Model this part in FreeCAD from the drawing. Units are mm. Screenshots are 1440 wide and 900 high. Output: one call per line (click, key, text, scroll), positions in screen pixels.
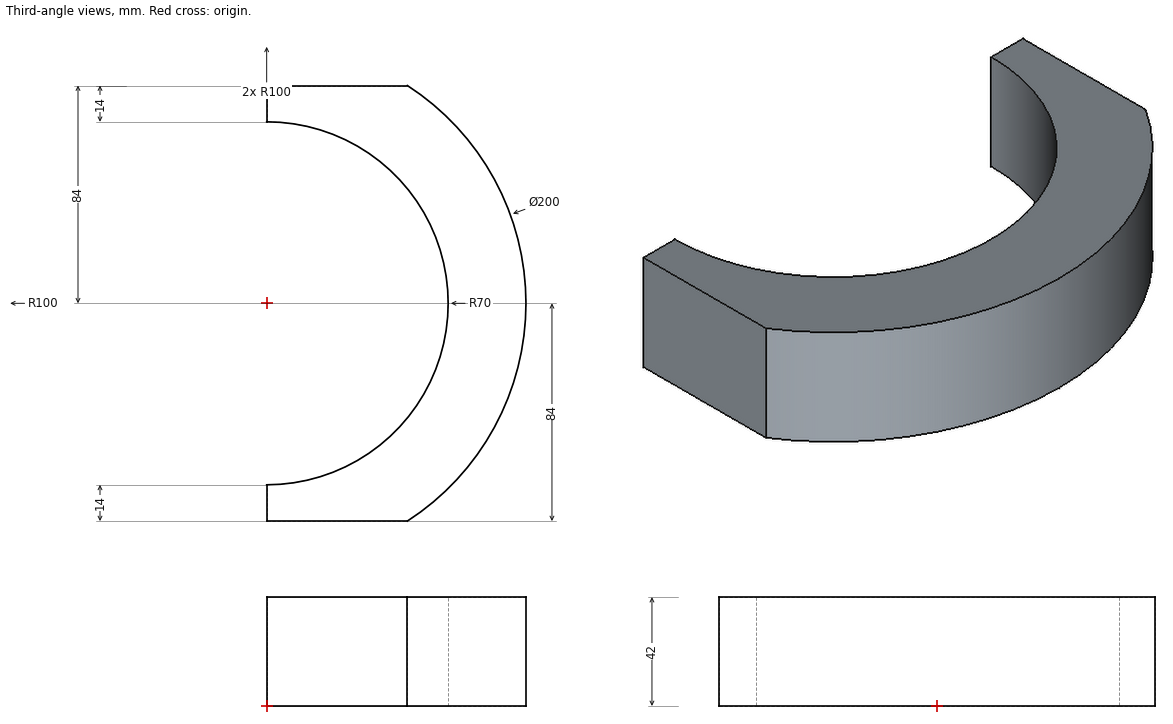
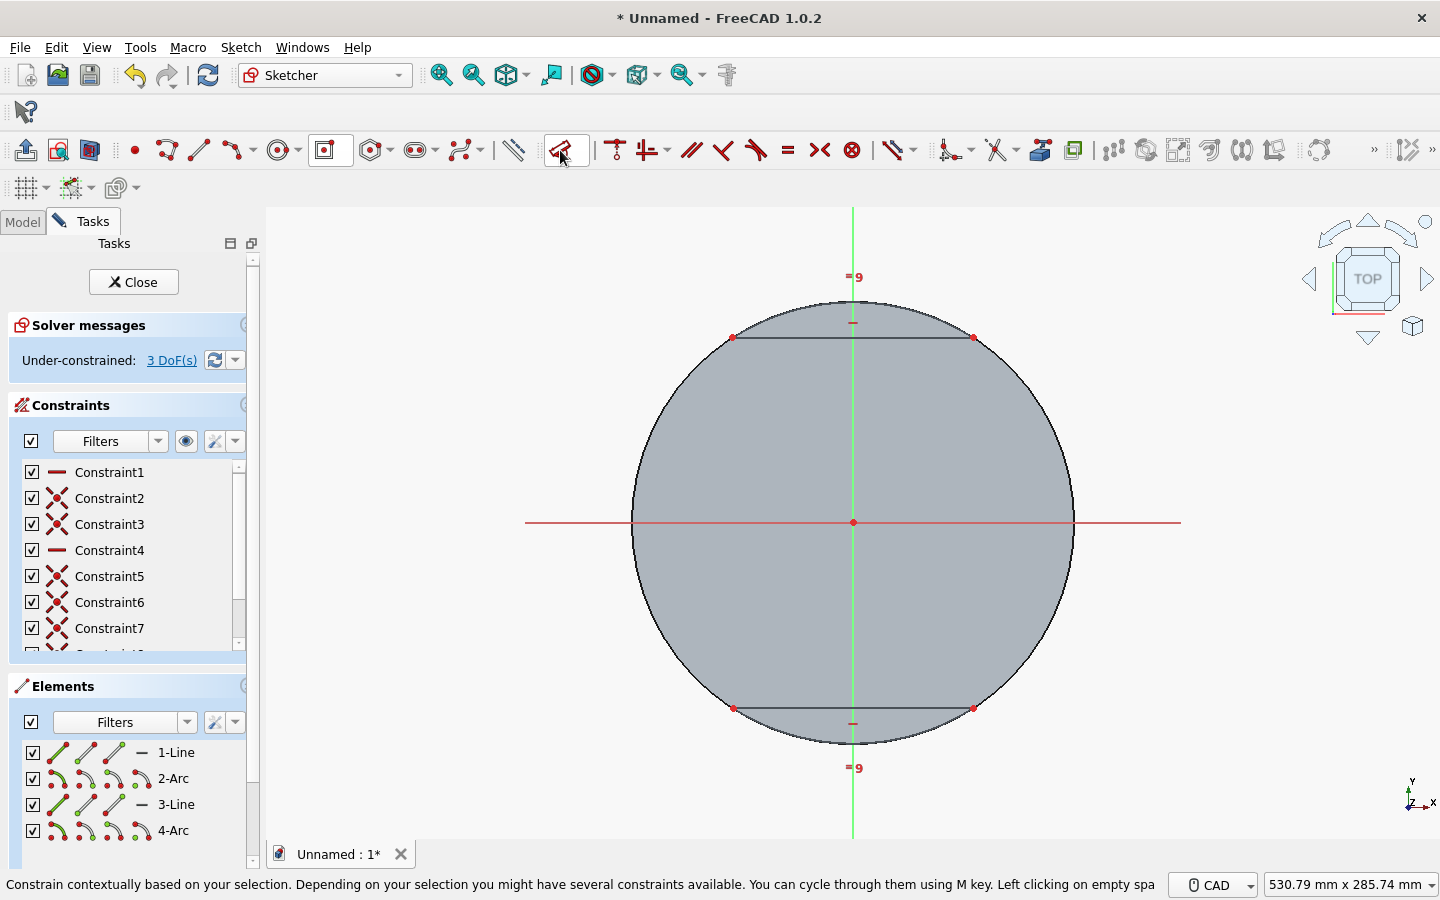
click(903, 308)
click(910, 277)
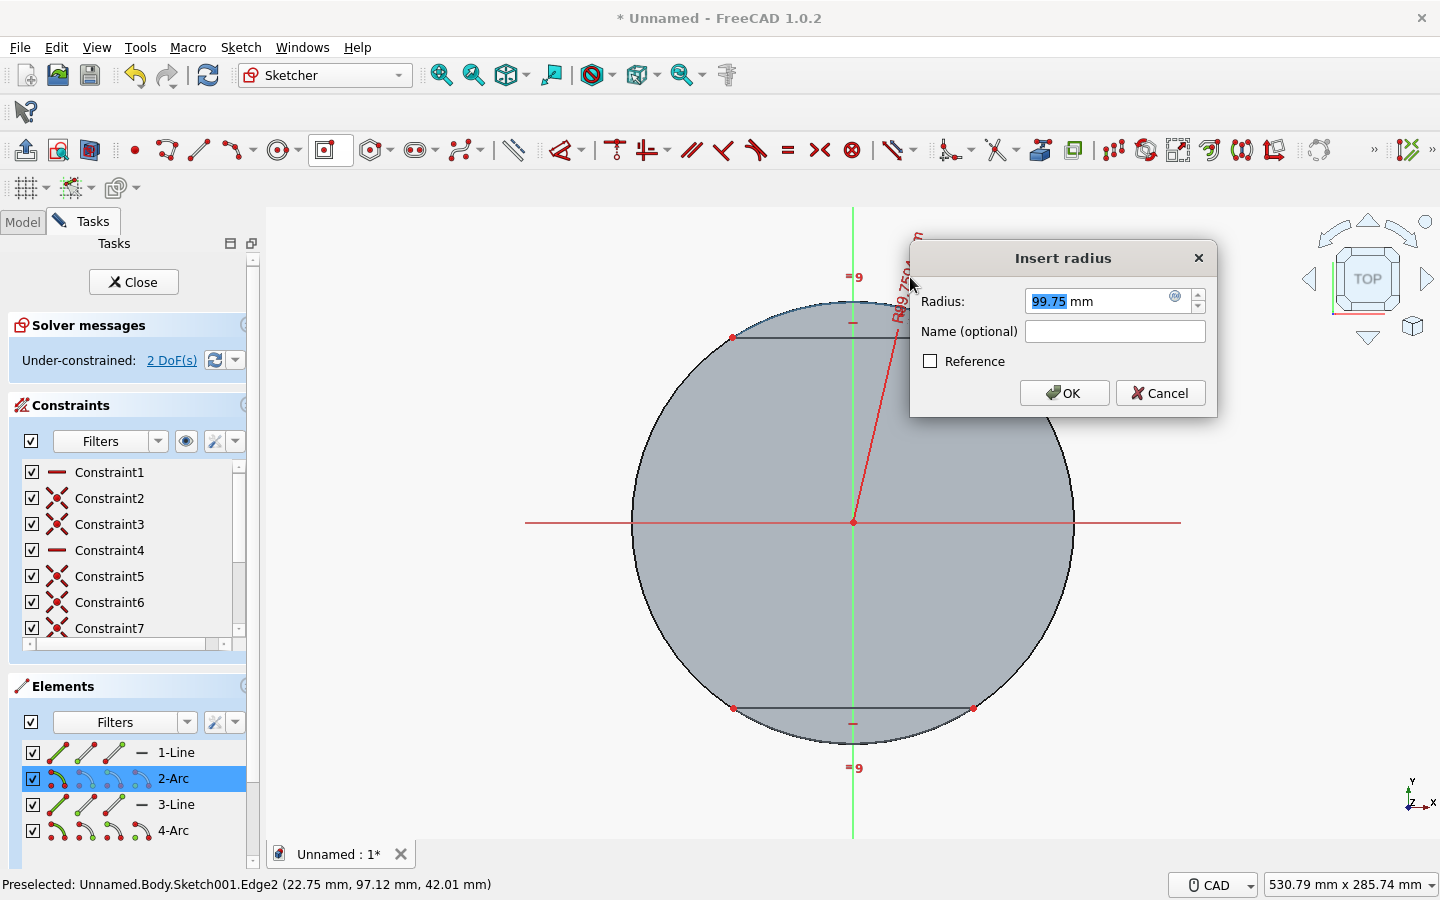
text(100)
key(Return)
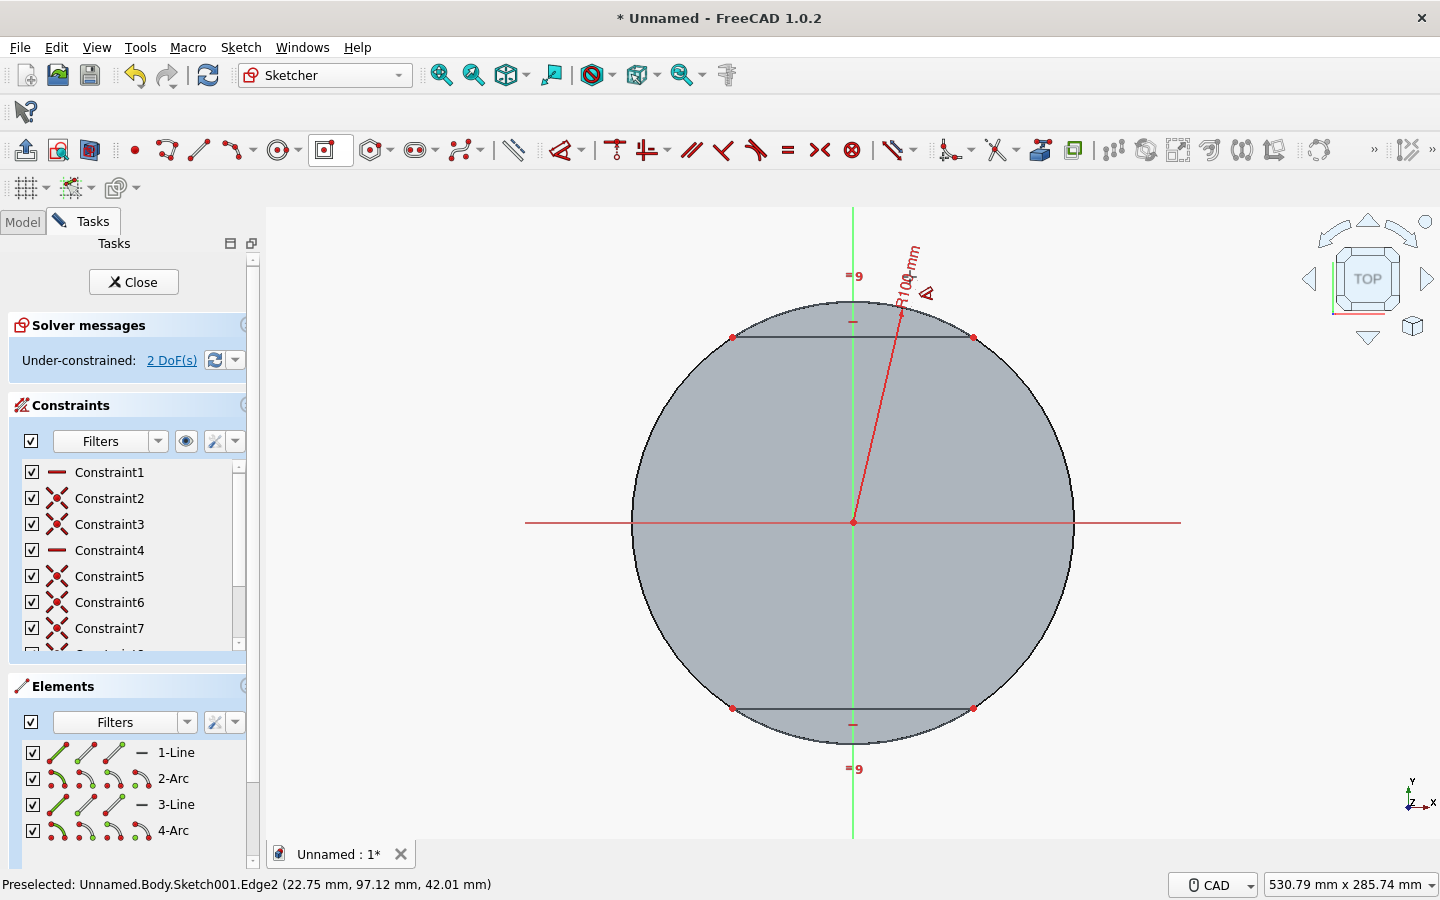
click(733, 337)
click(699, 430)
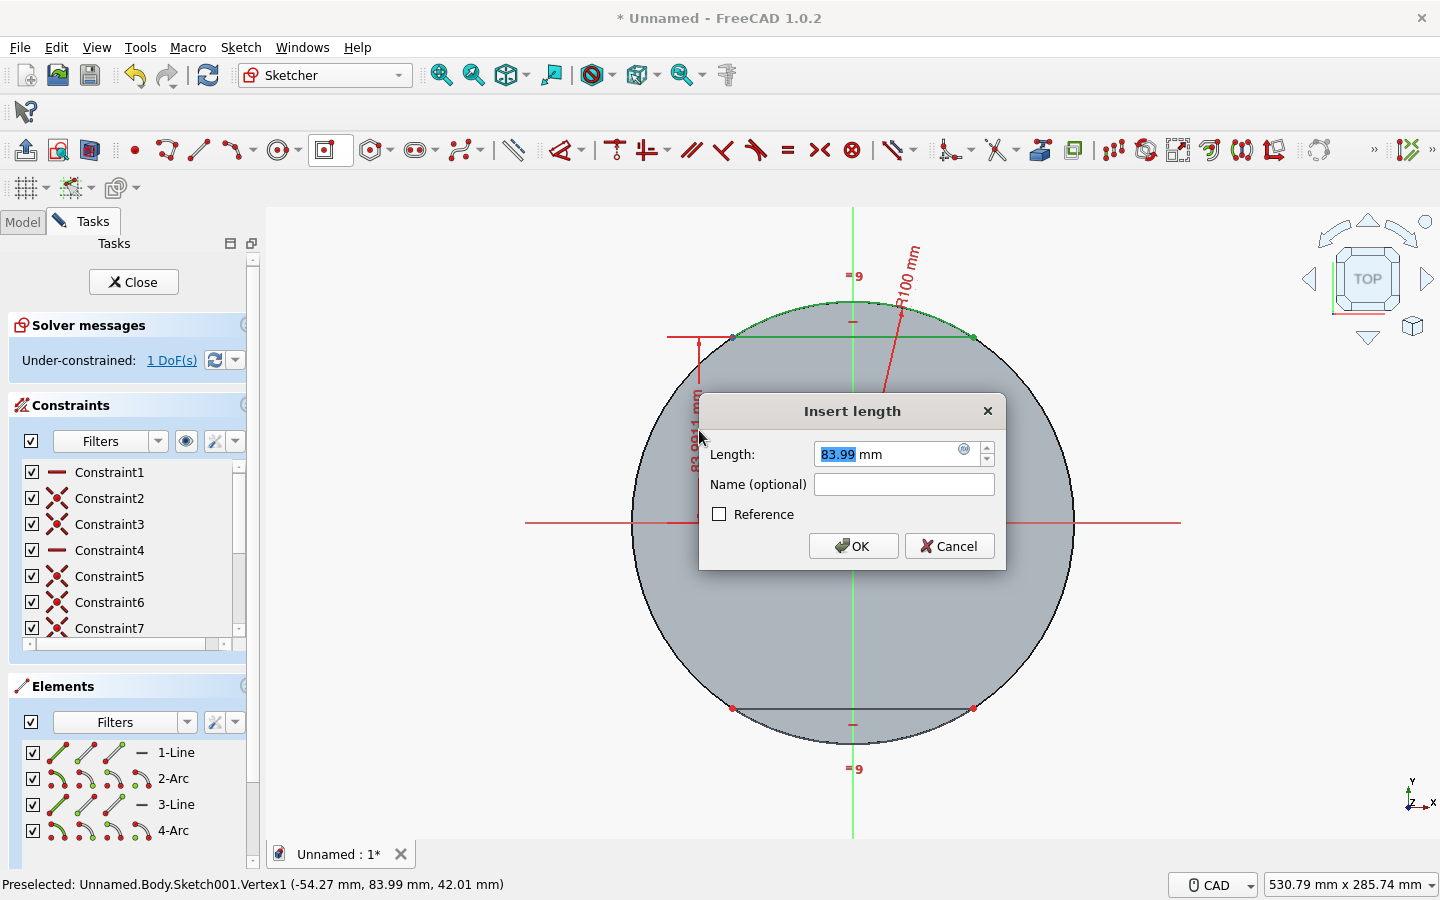
text(84)
key(Return)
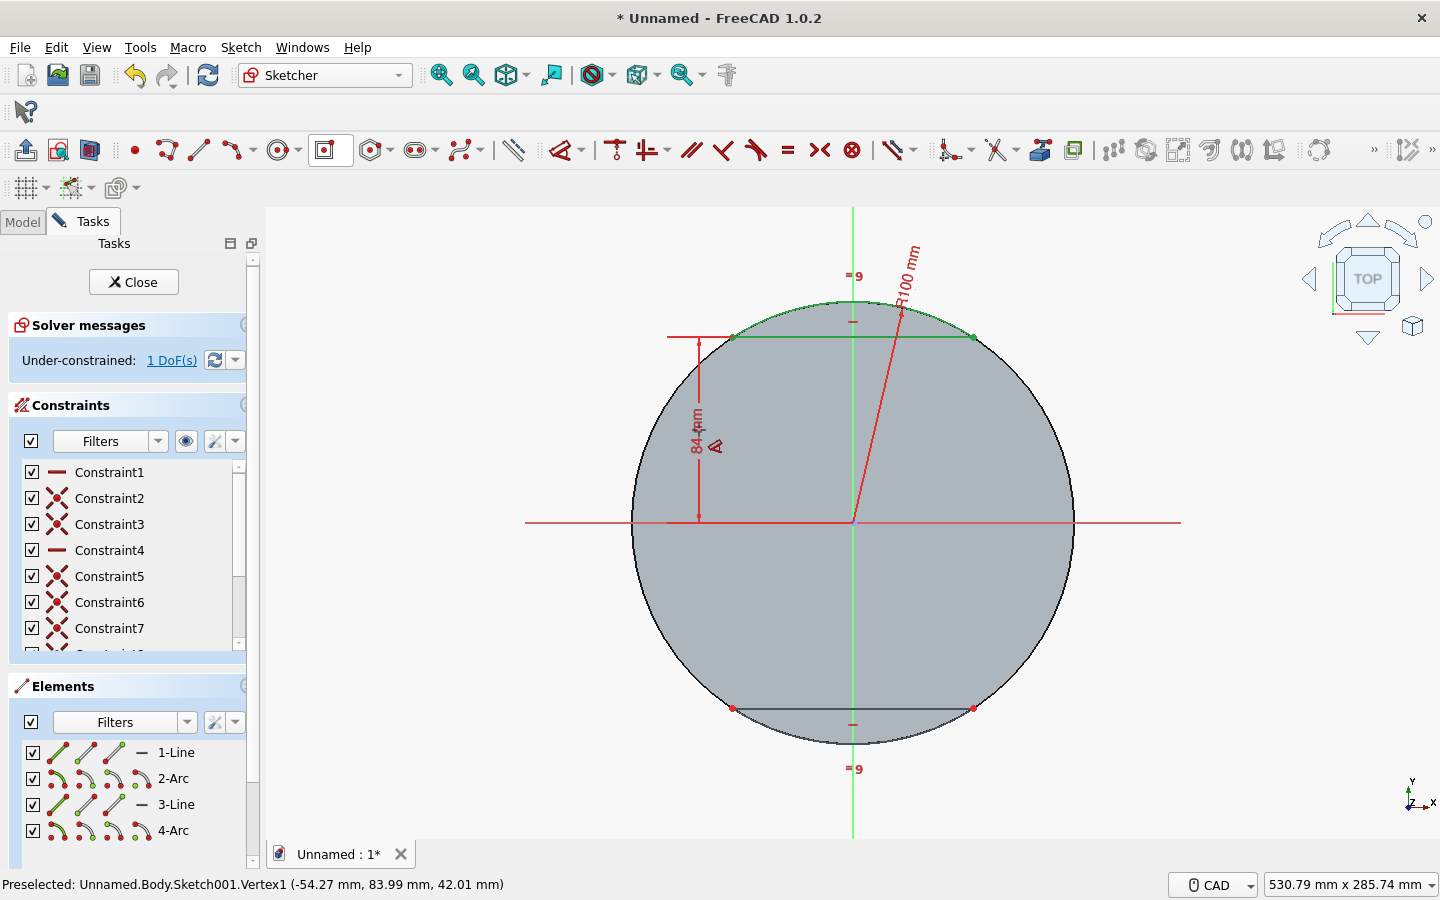
click(973, 709)
click(1007, 616)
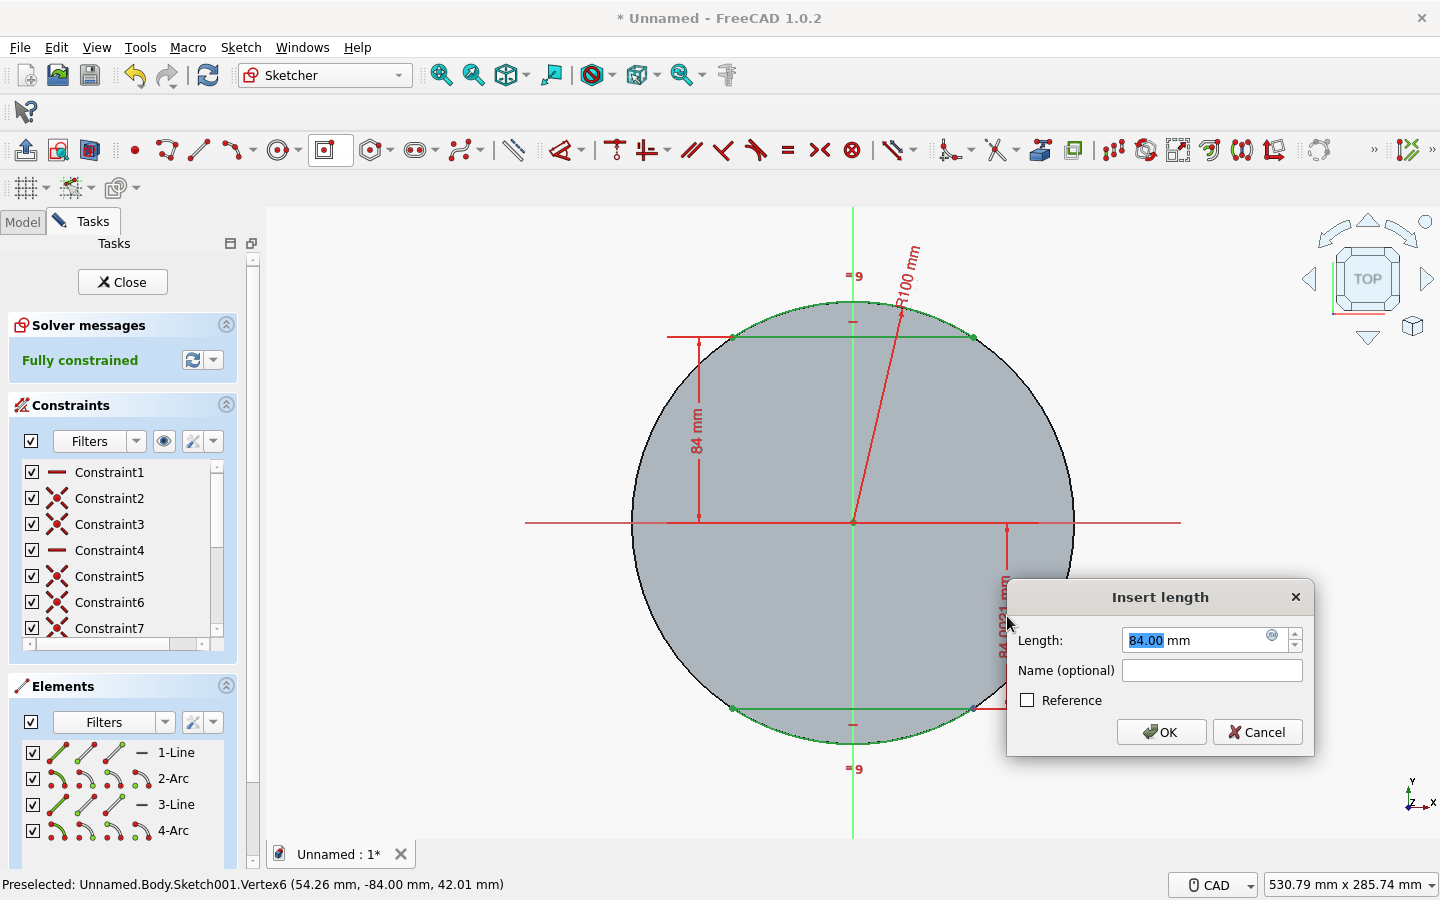
text(84)
key(Return)
key(Escape)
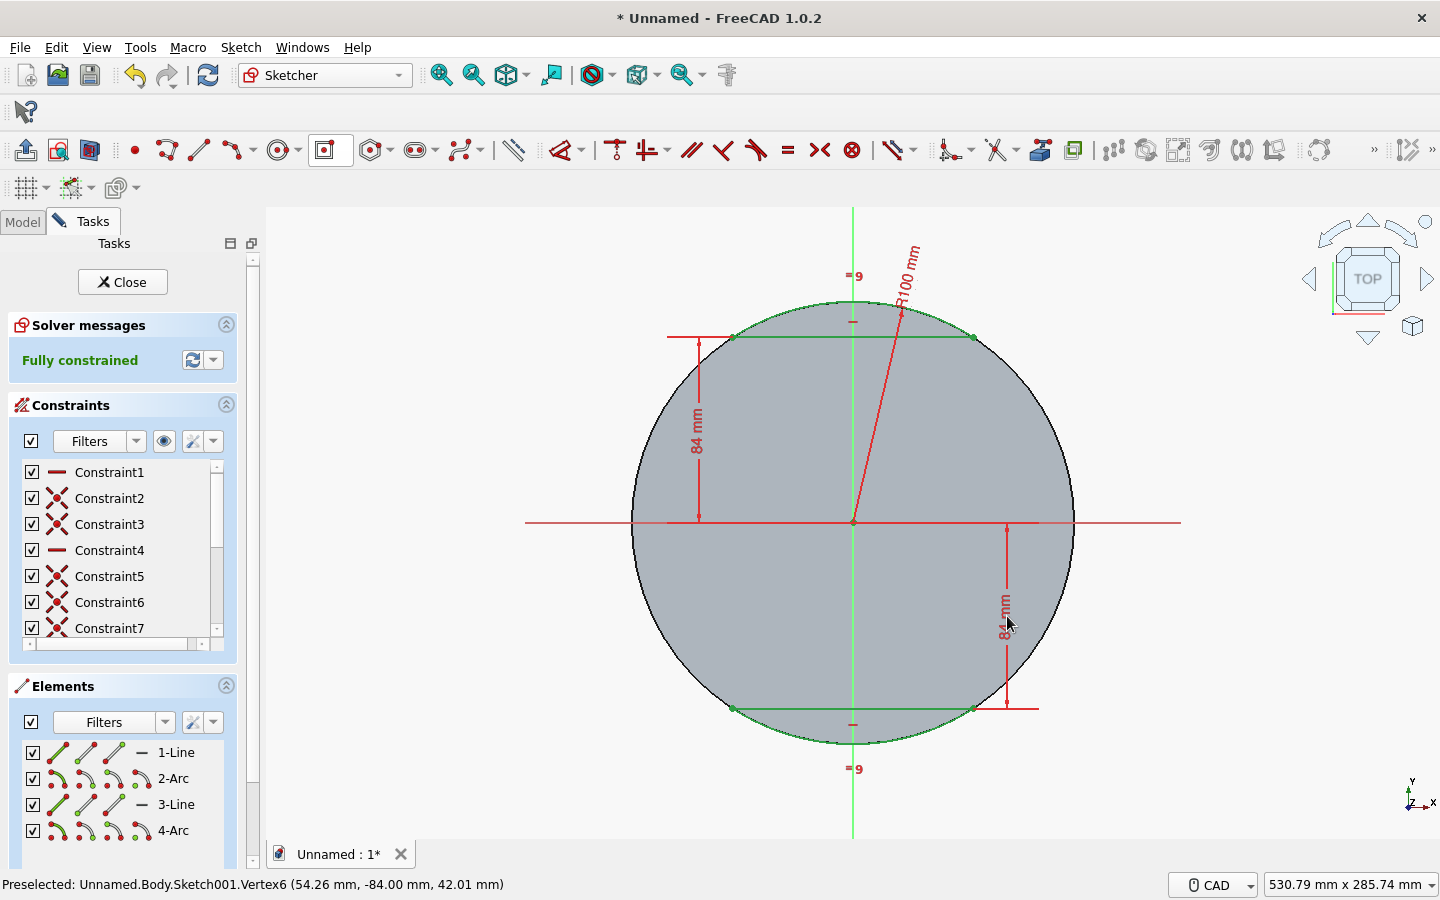
click(123, 282)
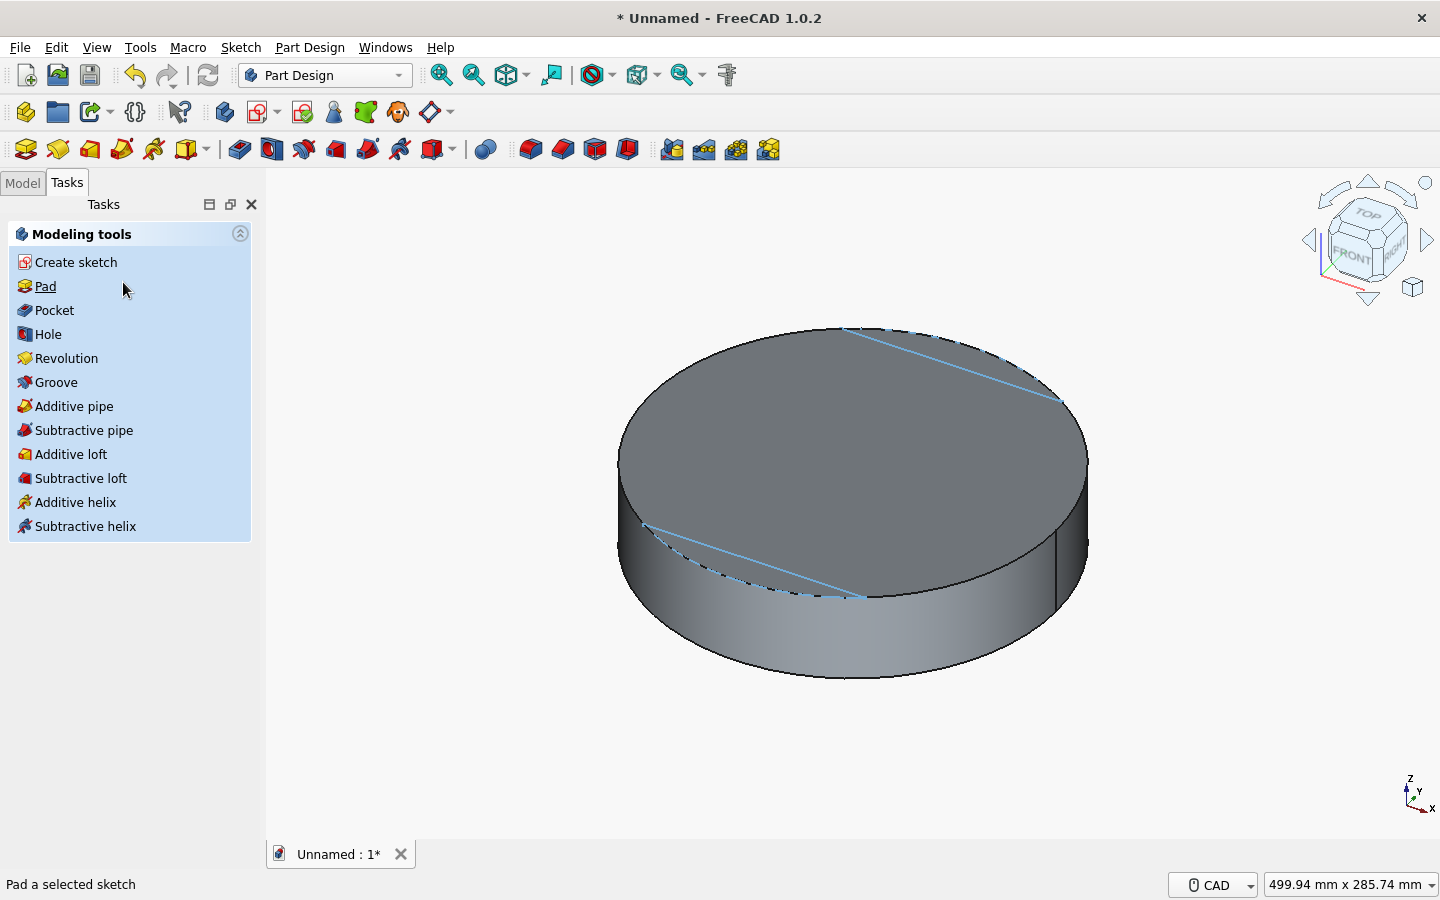
click(240, 150)